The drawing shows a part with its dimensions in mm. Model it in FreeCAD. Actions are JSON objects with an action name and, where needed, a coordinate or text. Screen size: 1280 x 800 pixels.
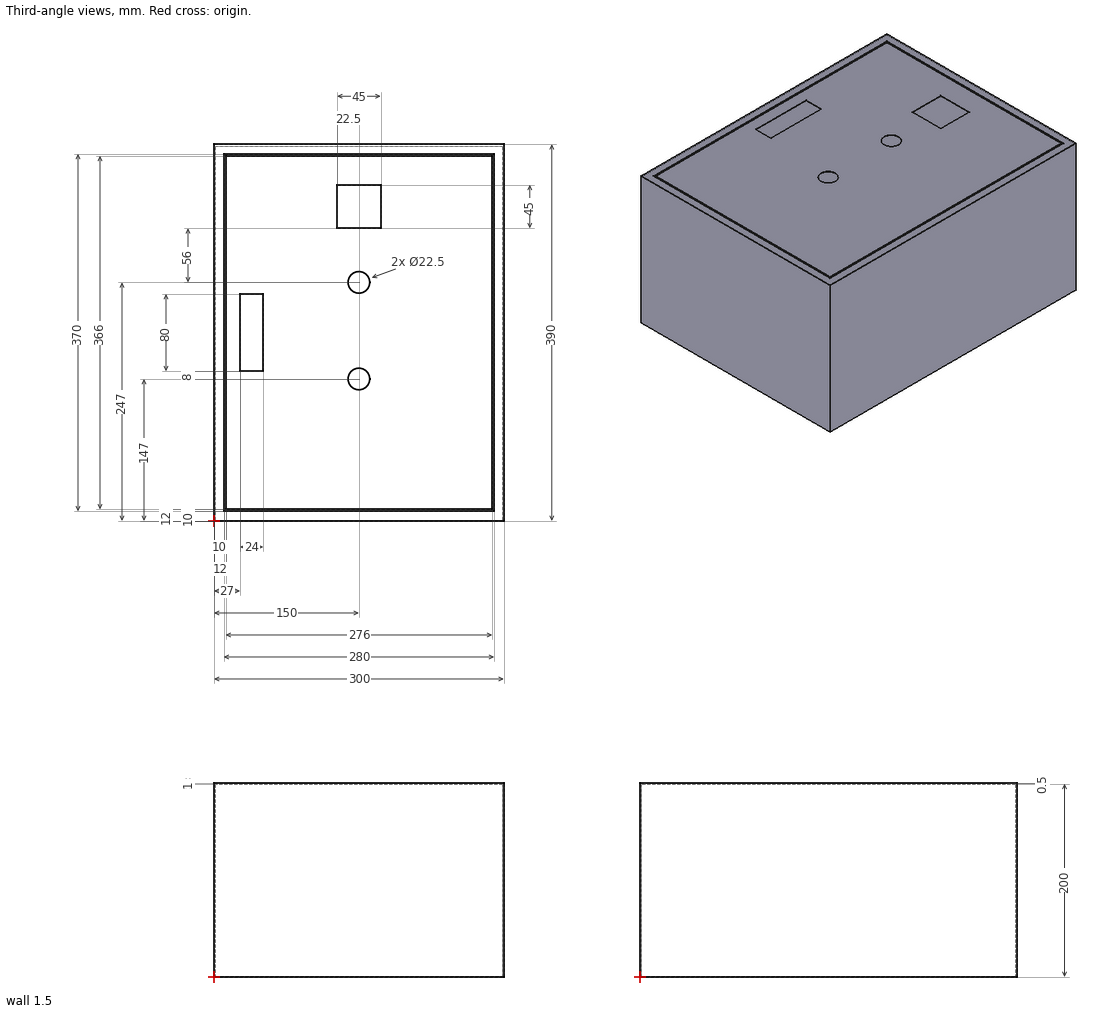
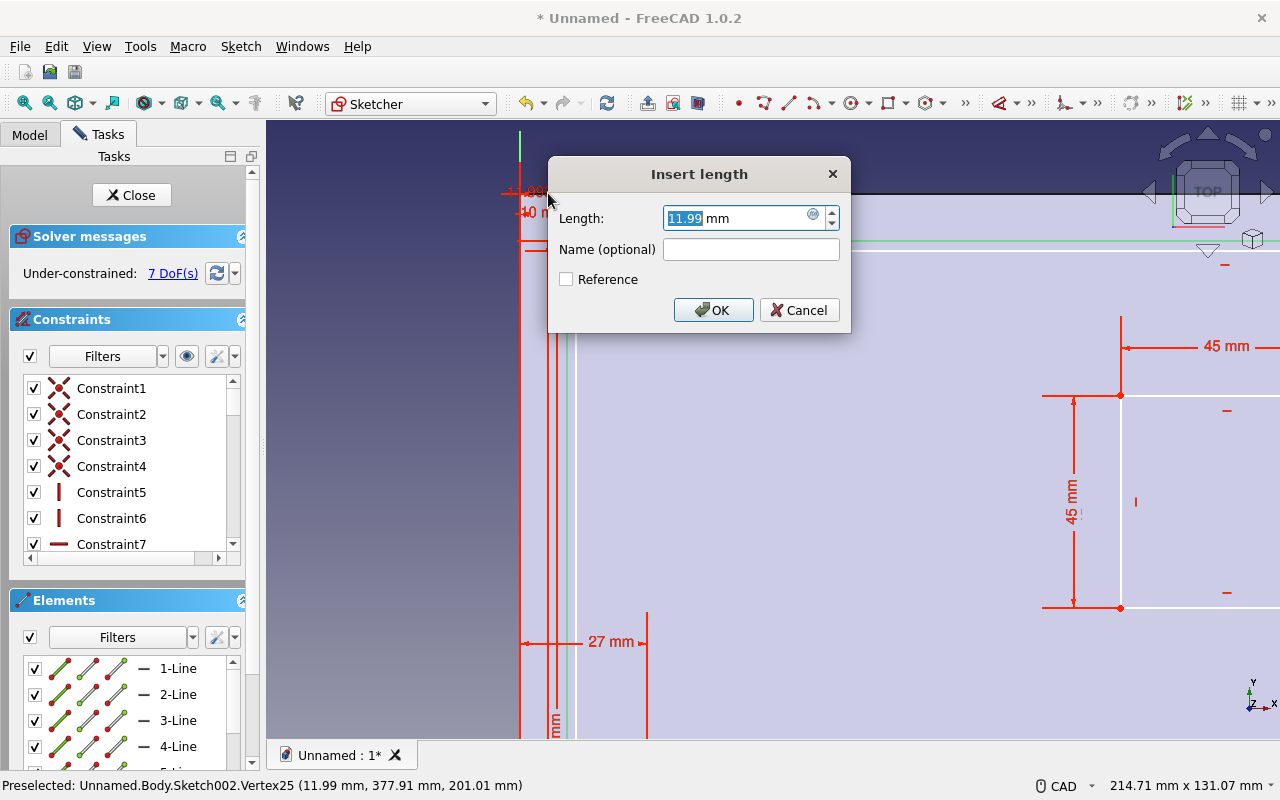
{"action": "type", "text": "12"}
{"action": "key", "text": "Return"}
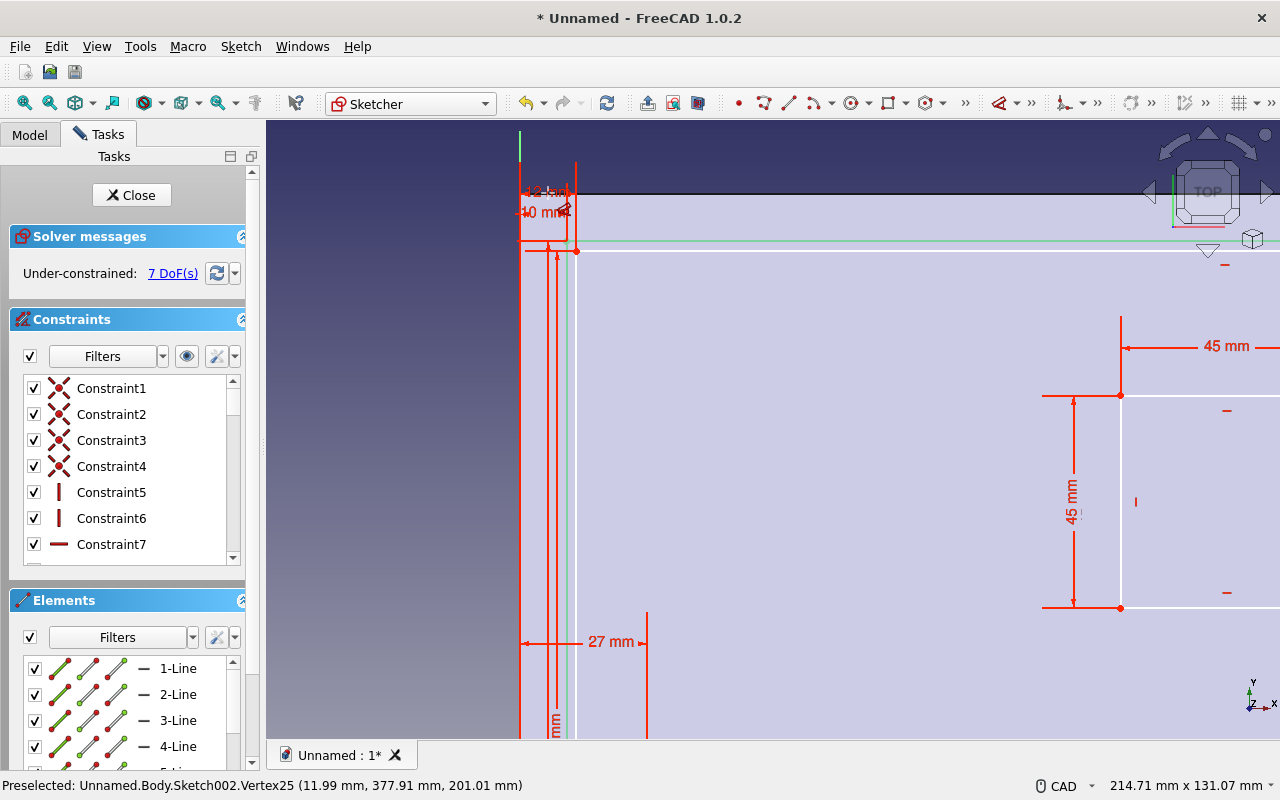
{"action": "scroll", "coordinate": [578, 250], "scroll_direction": "down", "scroll_amount": 8}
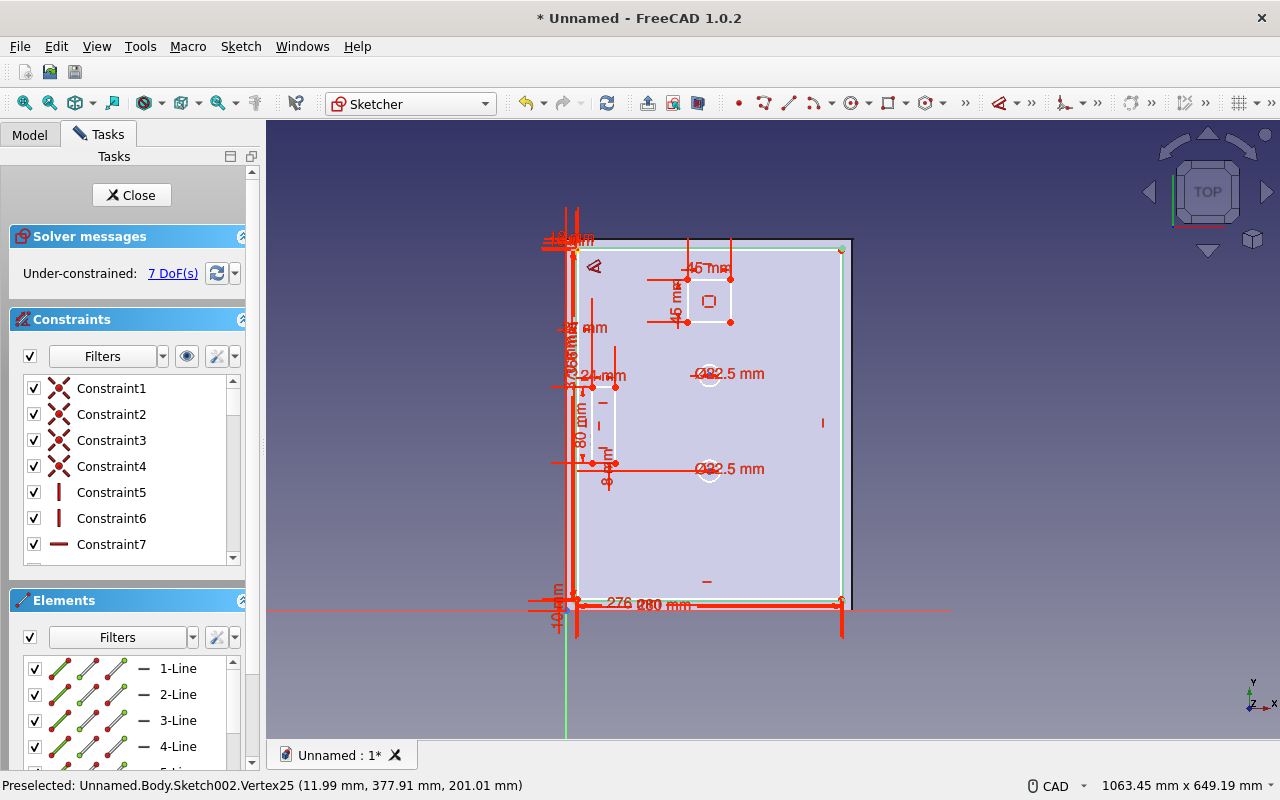
{"action": "scroll", "coordinate": [578, 599], "scroll_direction": "up", "scroll_amount": 8}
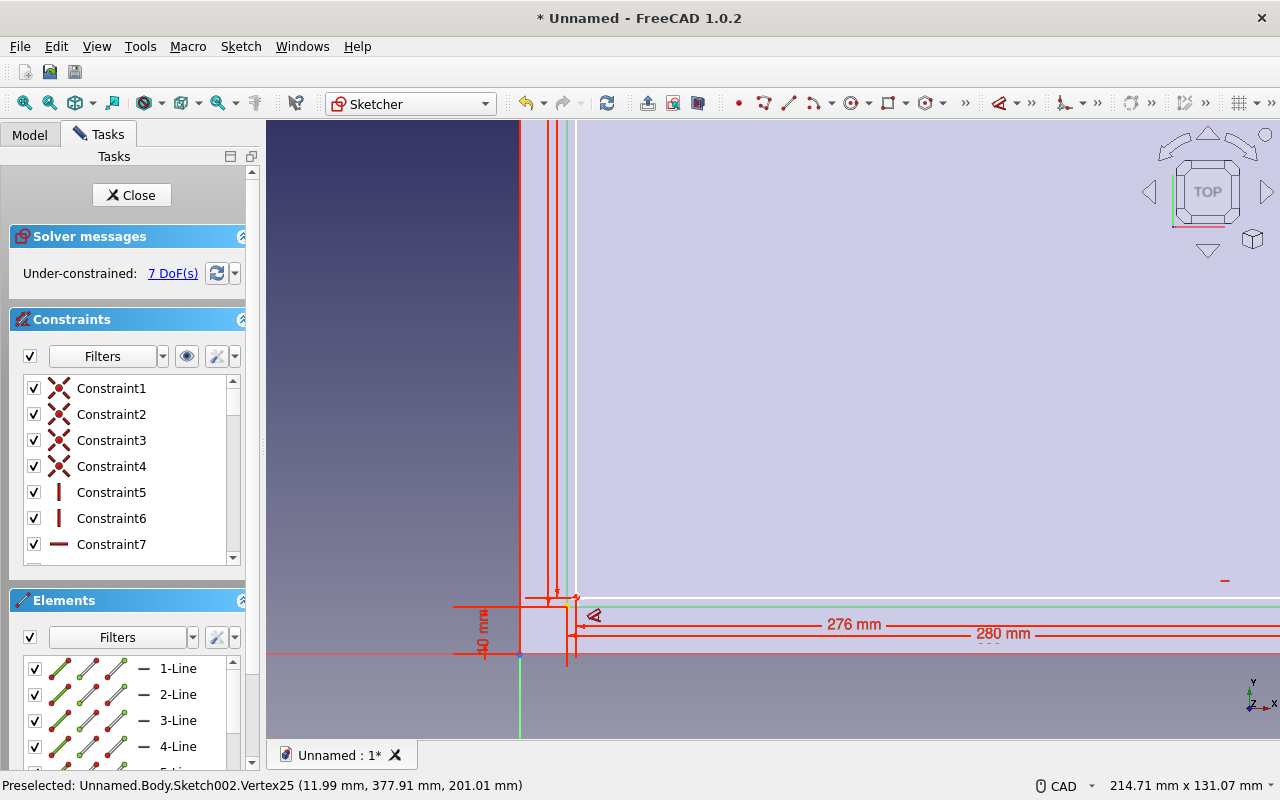
{"action": "left_click", "coordinate": [576, 598]}
{"action": "left_click", "coordinate": [486, 606]}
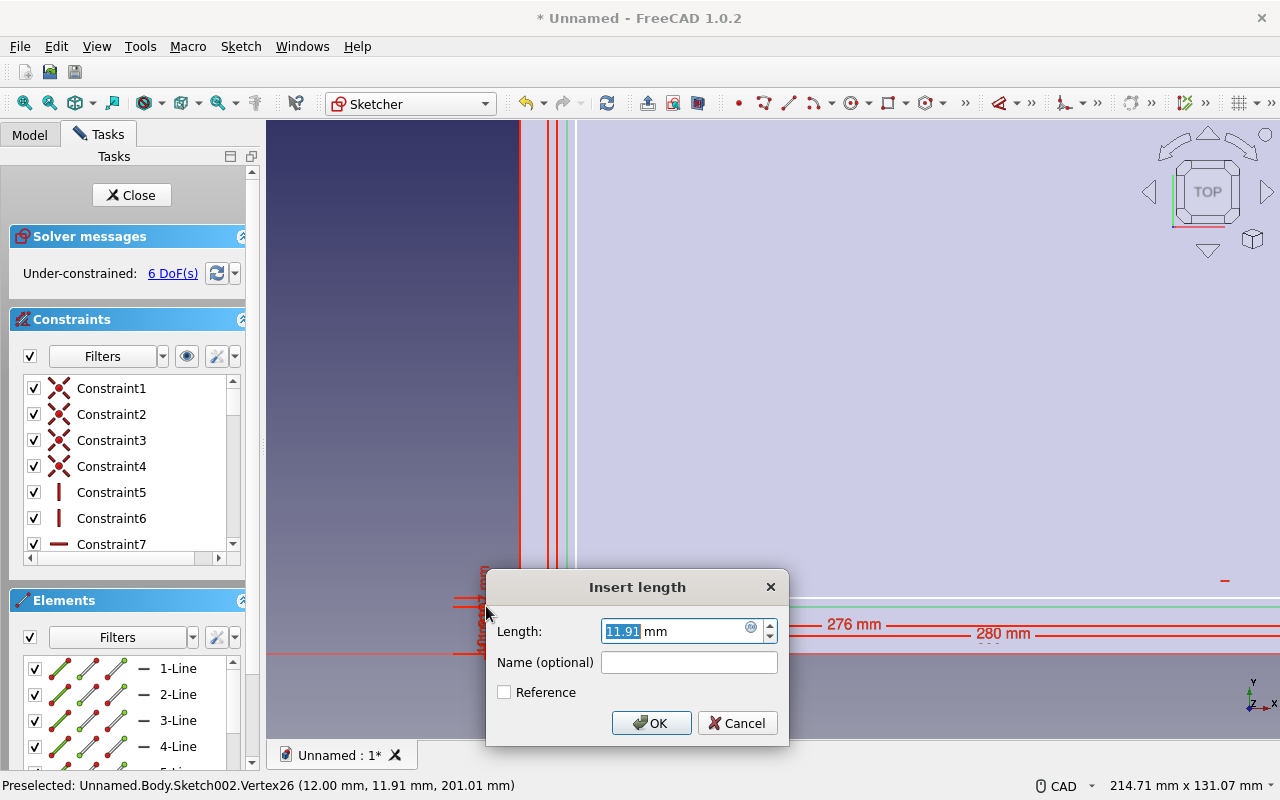
{"action": "type", "text": "12"}
{"action": "key", "text": "Return"}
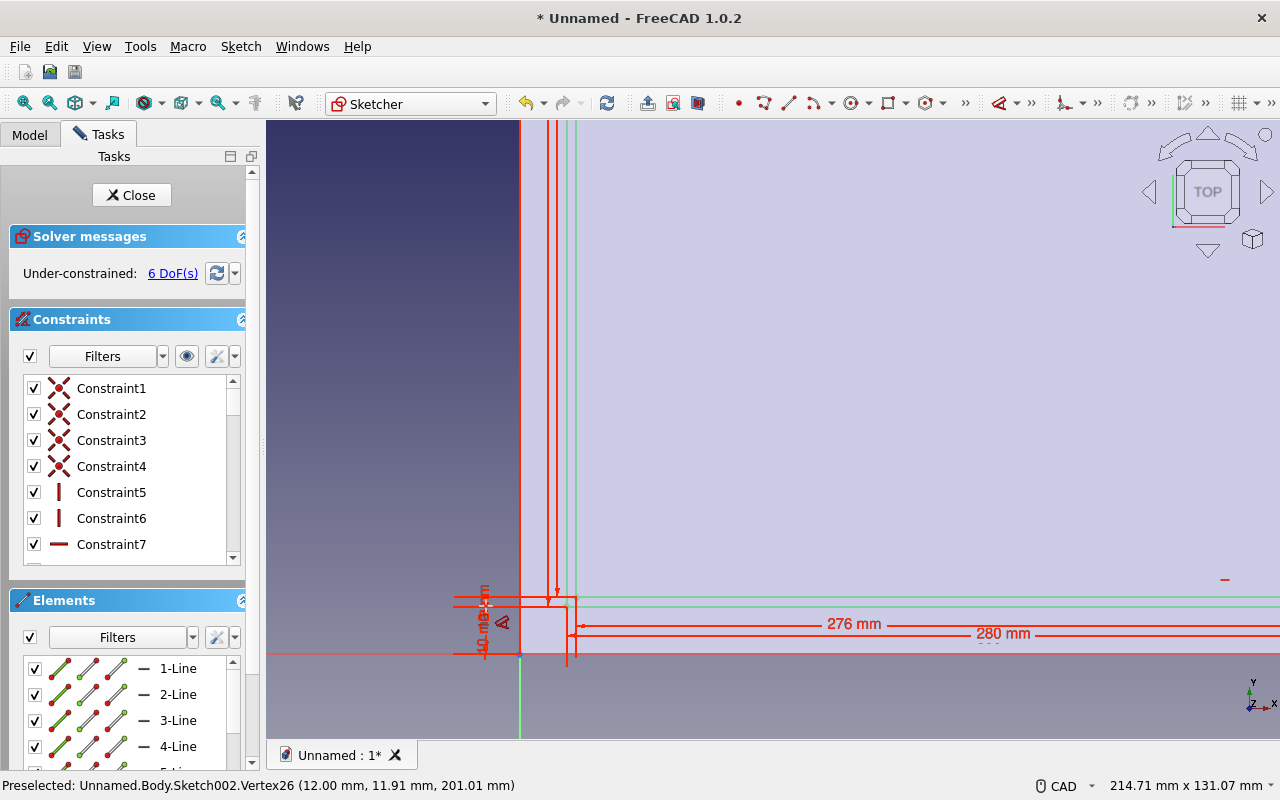
{"action": "scroll", "coordinate": [578, 600], "scroll_direction": "down", "scroll_amount": 8}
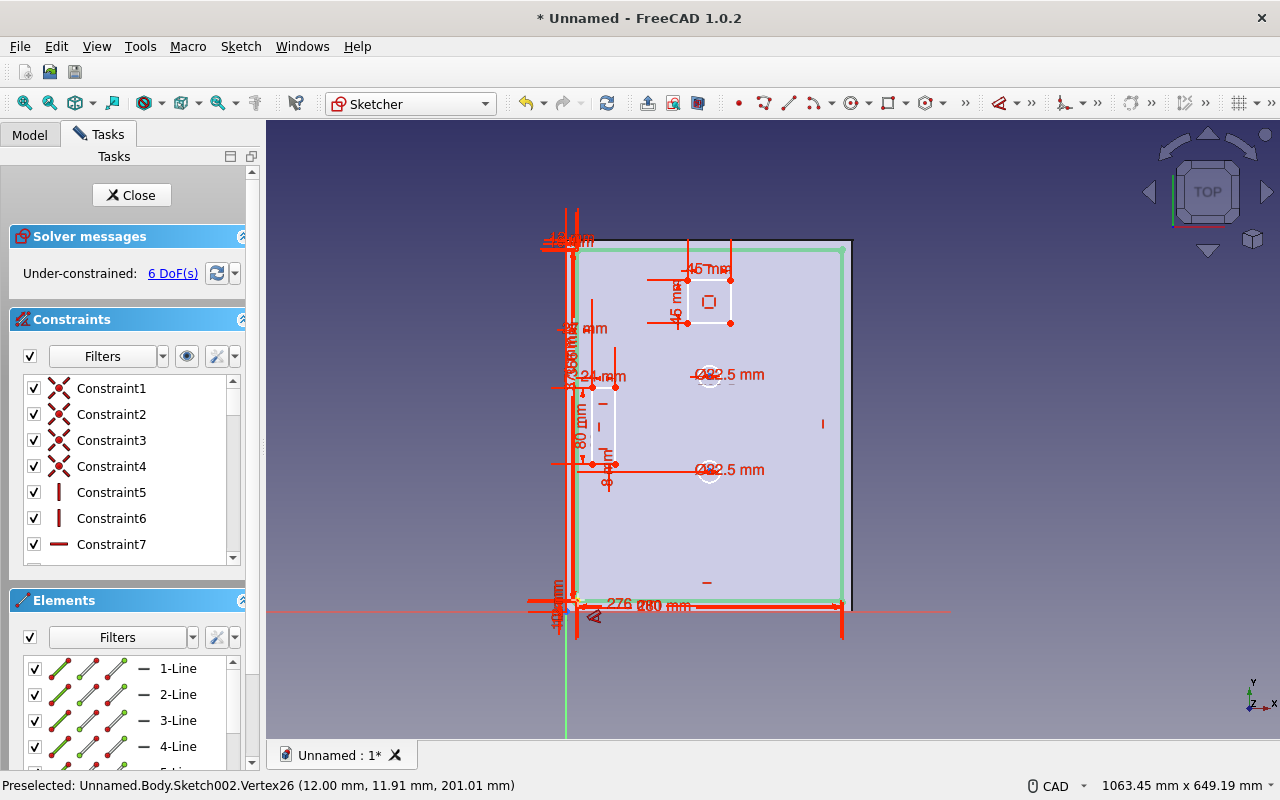
{"action": "left_click", "coordinate": [710, 377]}
{"action": "left_click", "coordinate": [638, 646]}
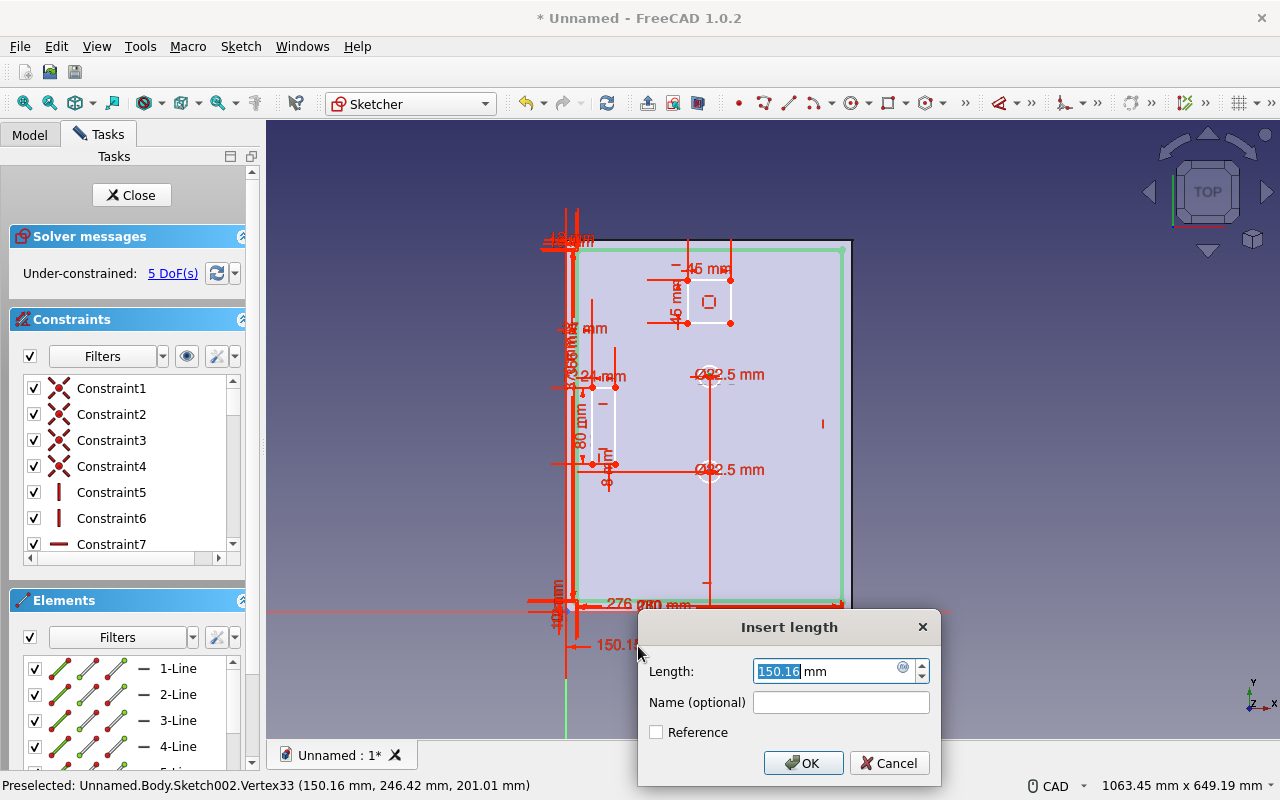
{"action": "type", "text": "150"}
{"action": "key", "text": "Return"}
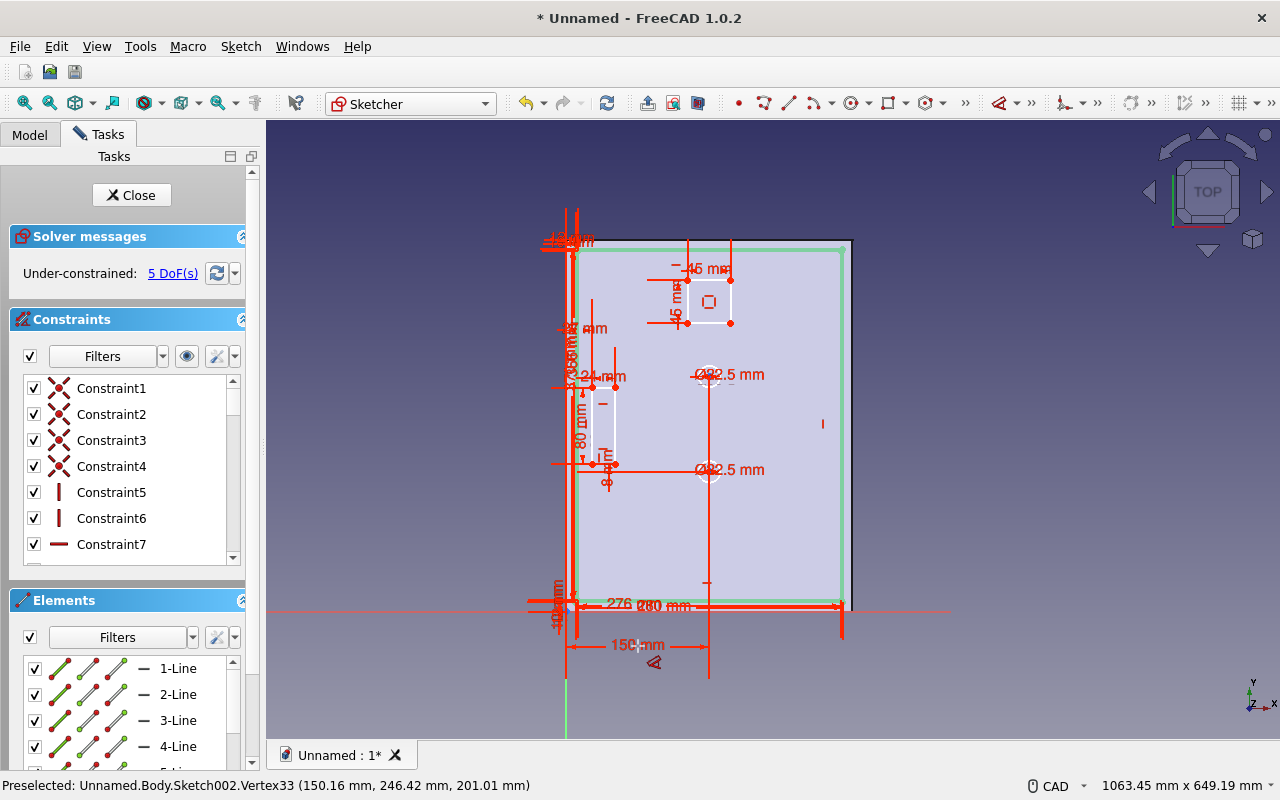
{"action": "left_click", "coordinate": [709, 377]}
{"action": "left_click", "coordinate": [532, 494]}